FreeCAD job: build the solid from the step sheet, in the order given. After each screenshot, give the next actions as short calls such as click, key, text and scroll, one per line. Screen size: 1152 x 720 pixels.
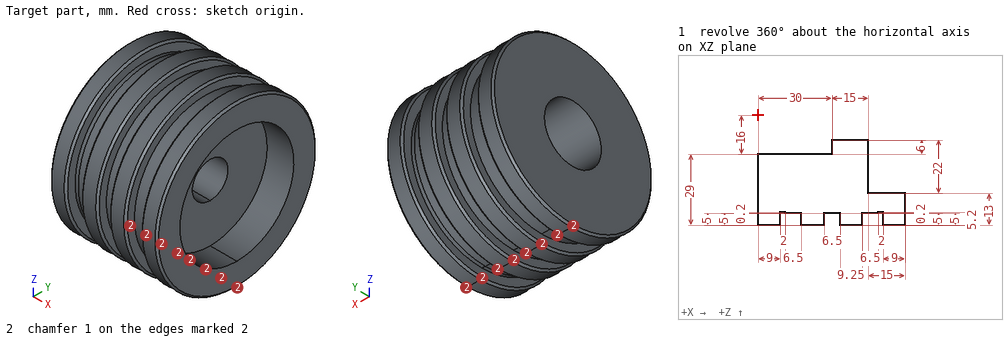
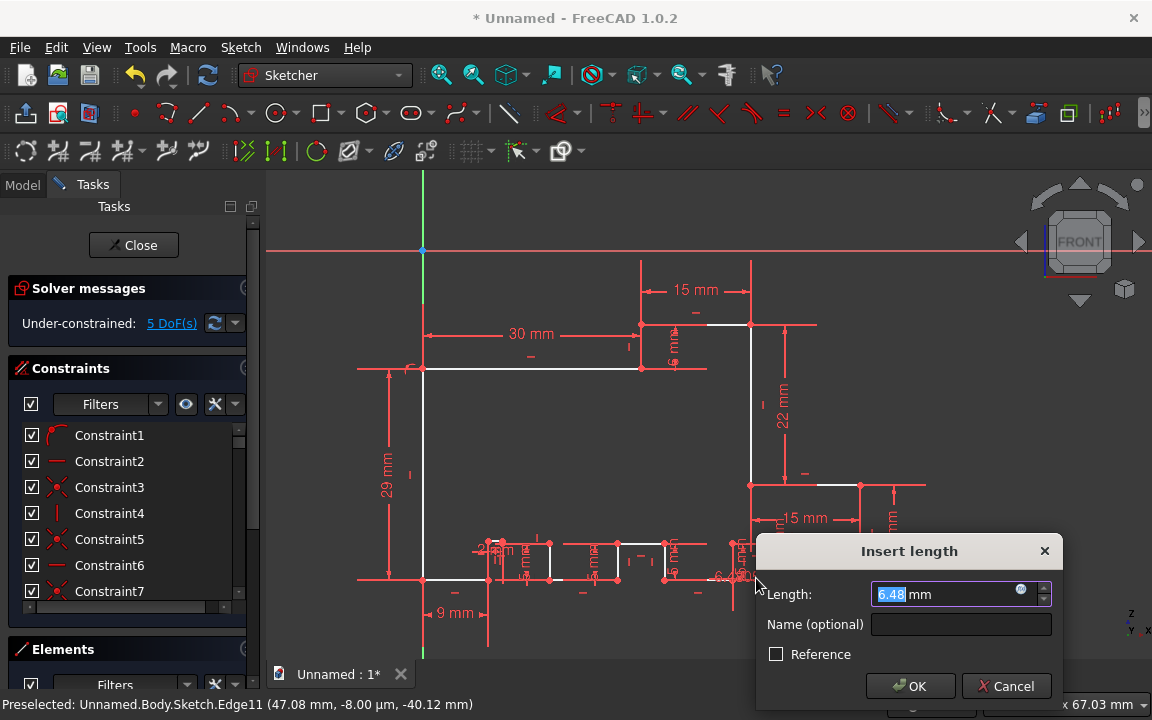
text(6.5)
key(Return)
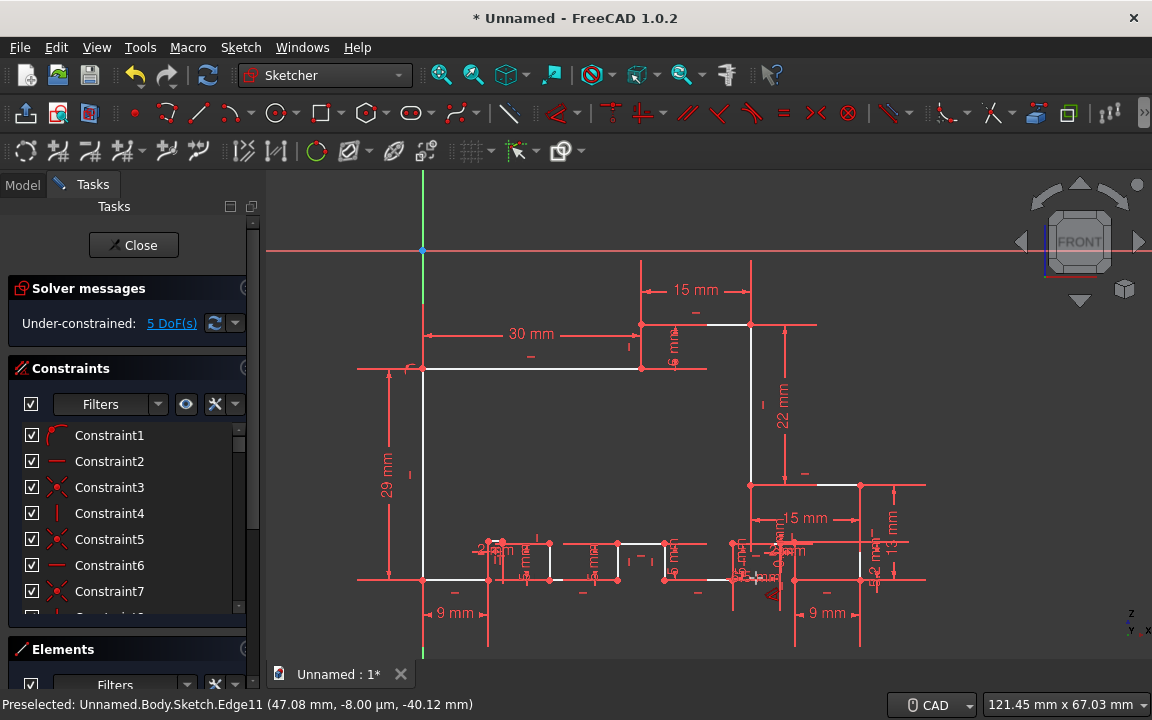
click(651, 544)
click(641, 510)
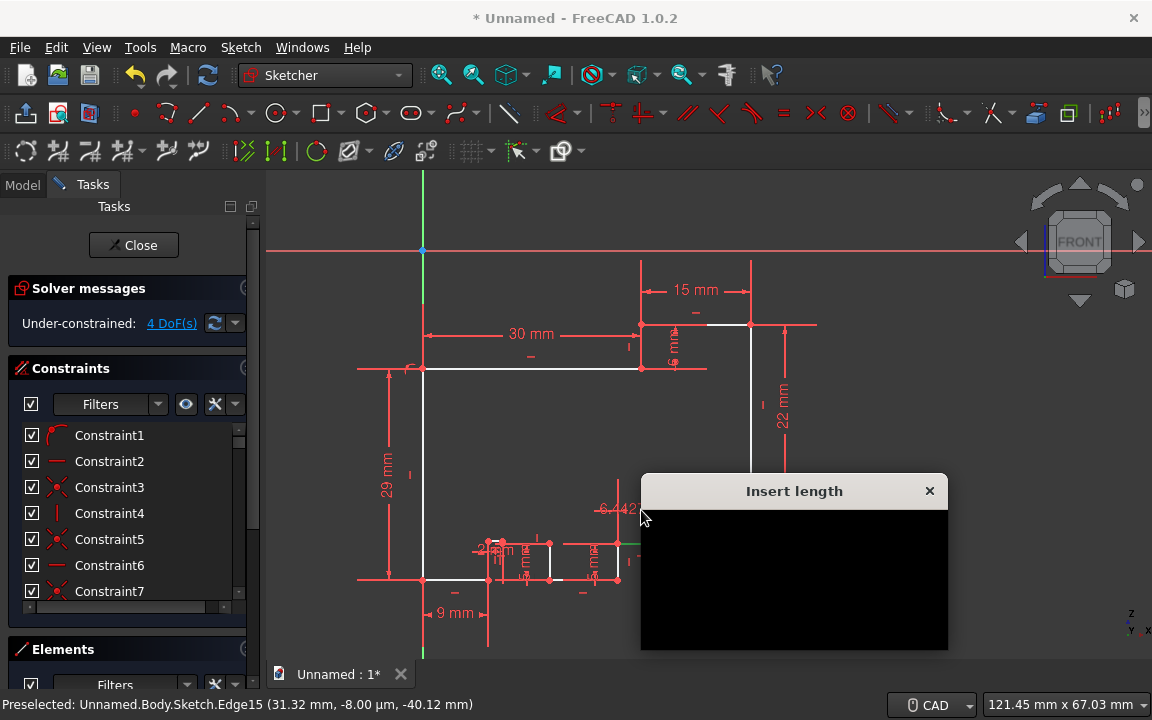
text(6.5)
key(Return)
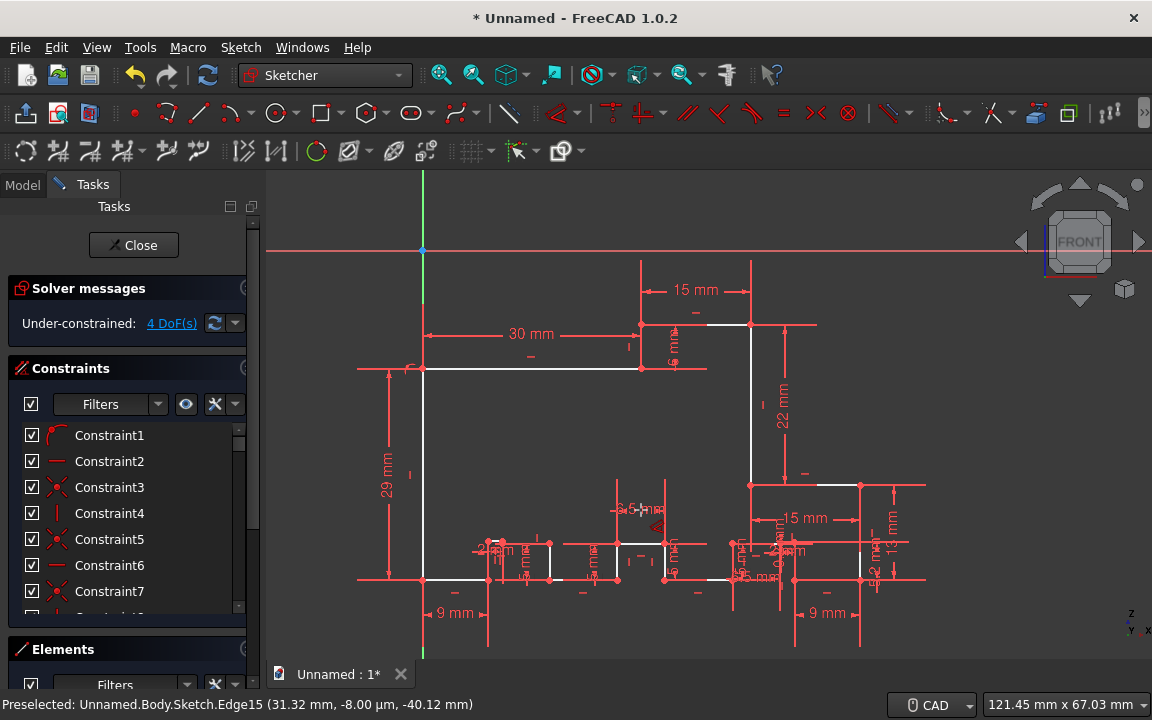
click(536, 544)
click(526, 510)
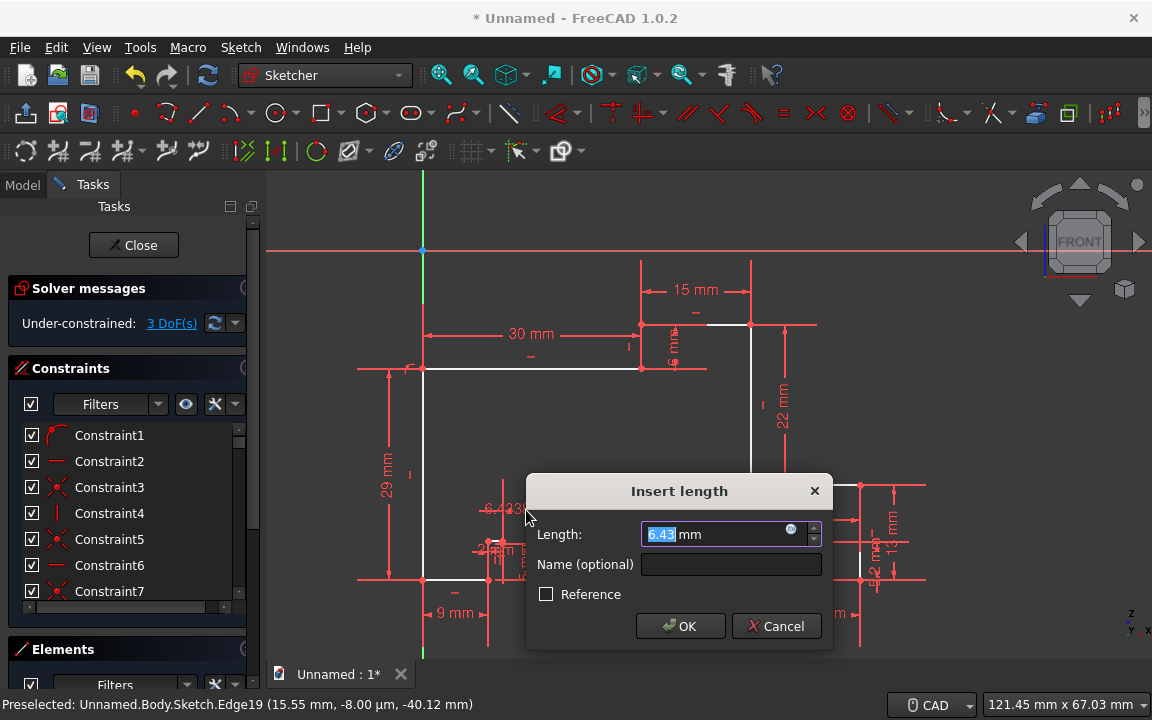
text(6.5)
key(Return)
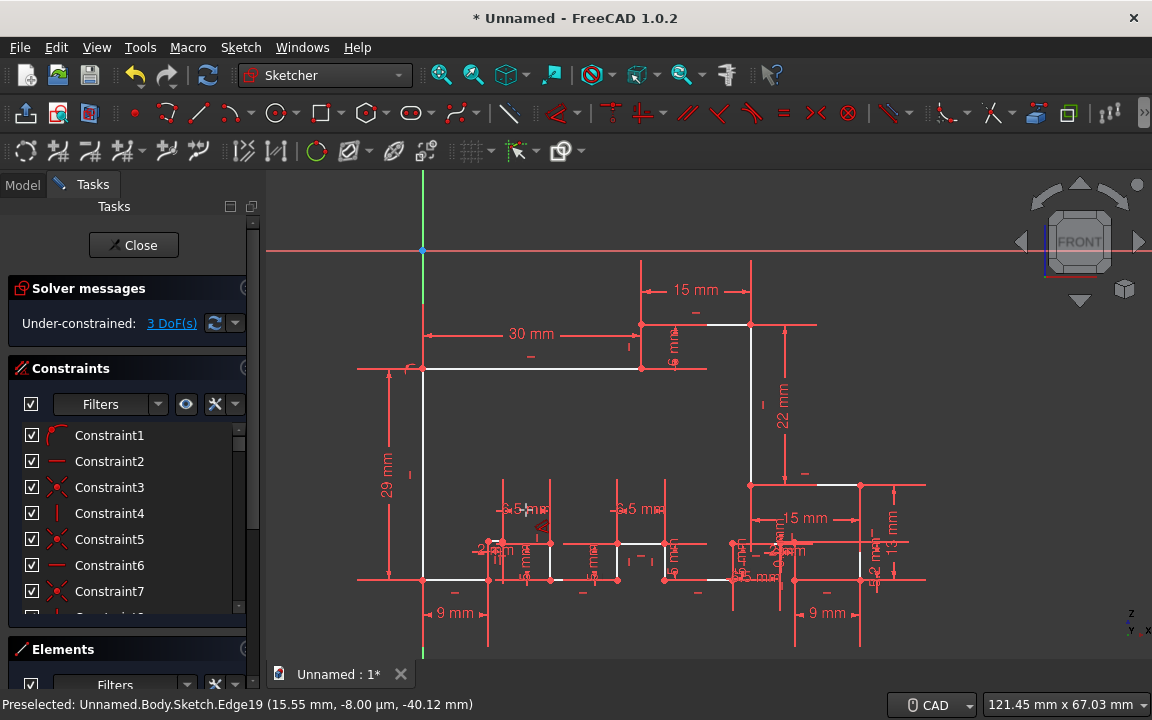
scroll(503, 542, up, 17)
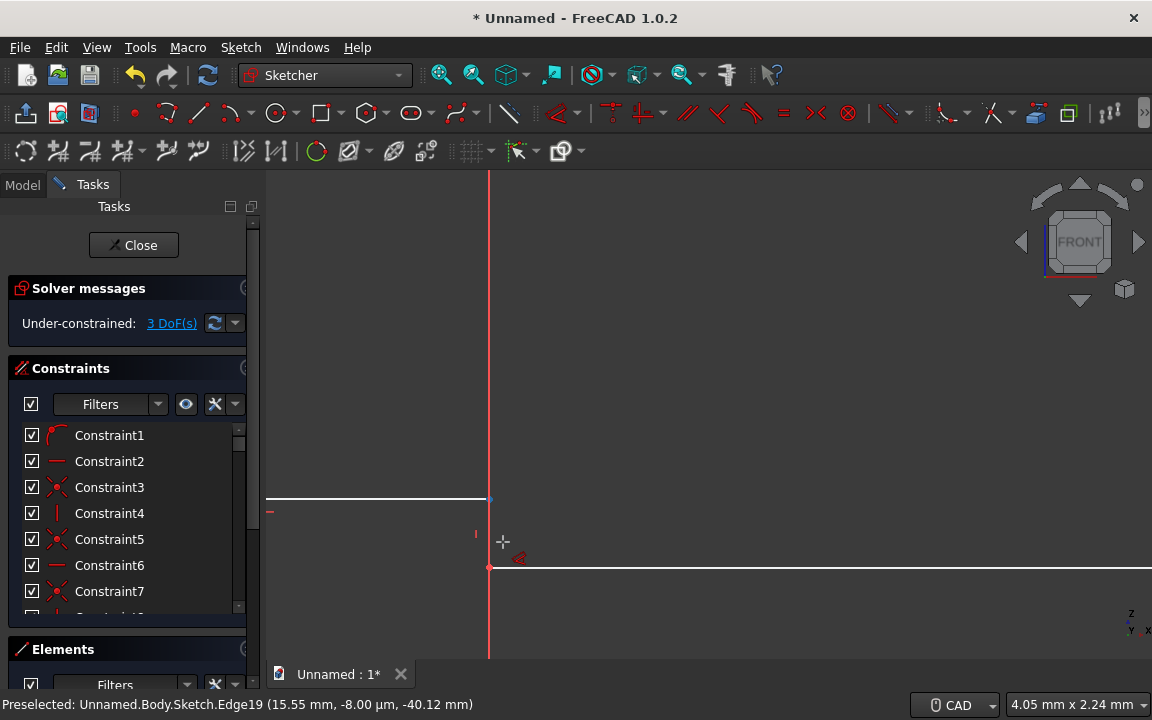
click(489, 533)
click(455, 533)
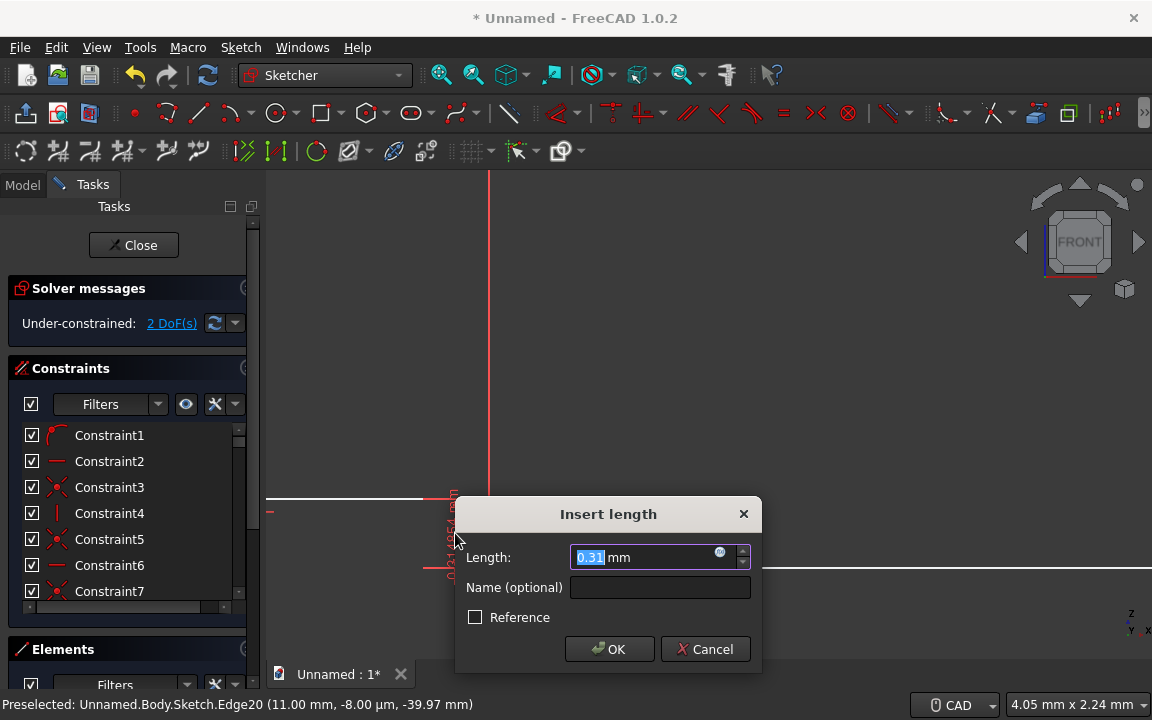
text(0.2)
key(Return)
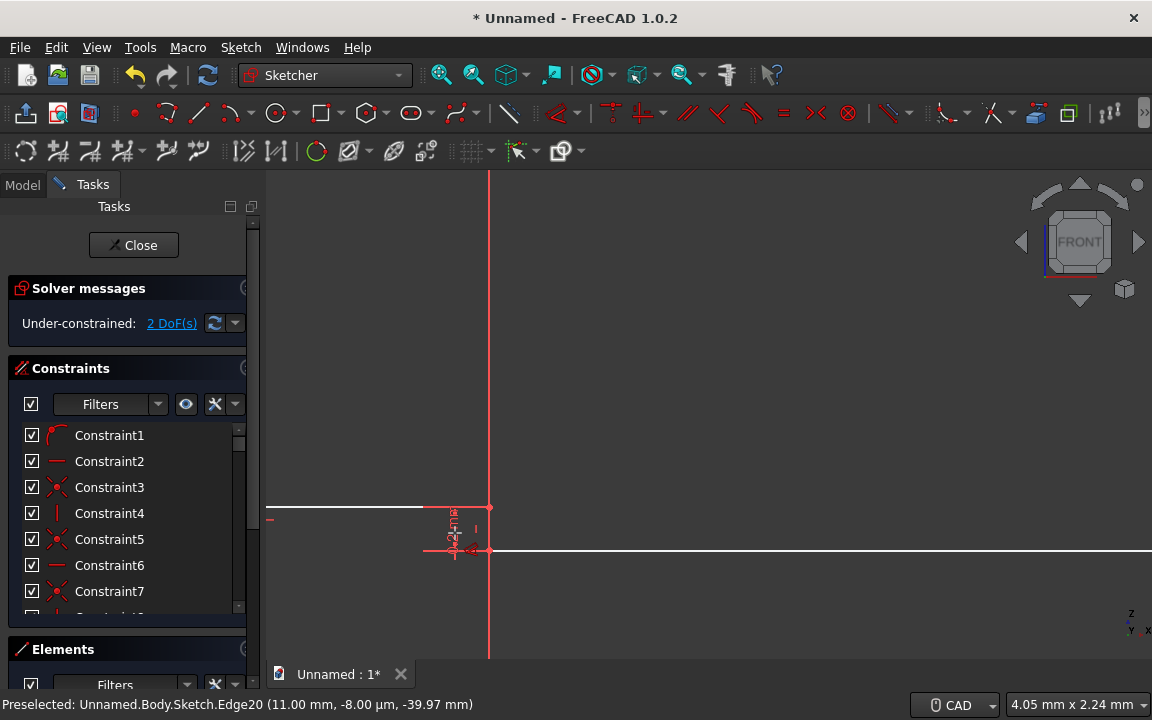
scroll(502, 542, down, 17)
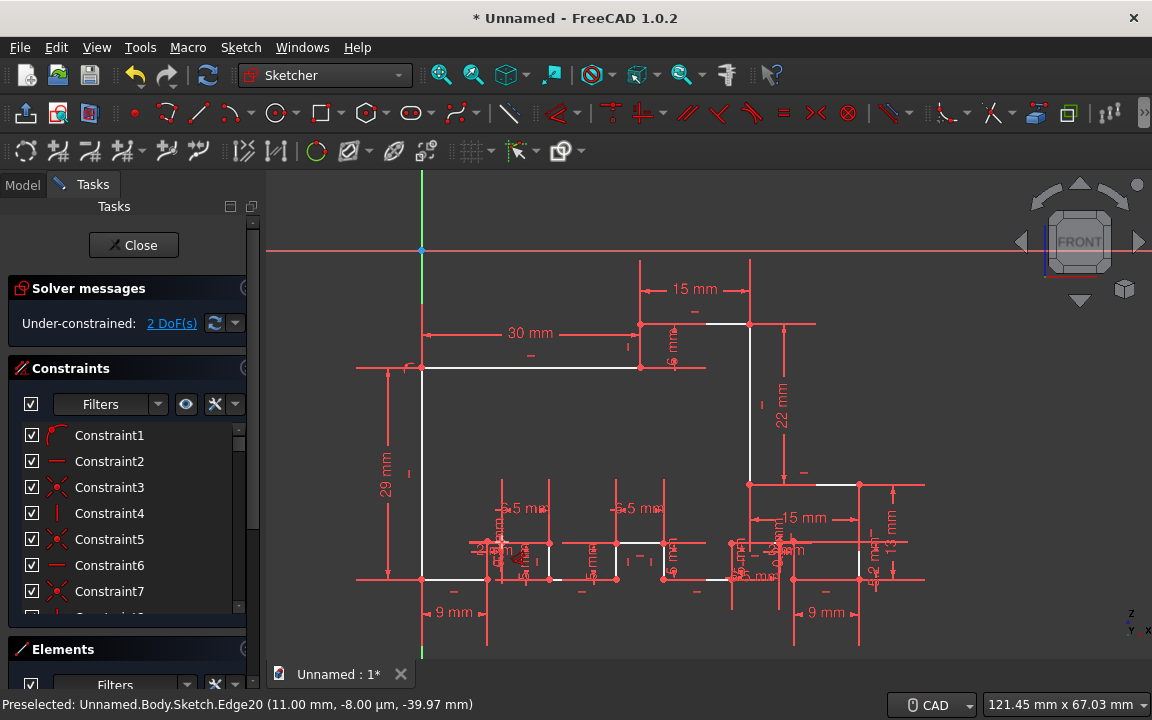
click(422, 368)
click(388, 309)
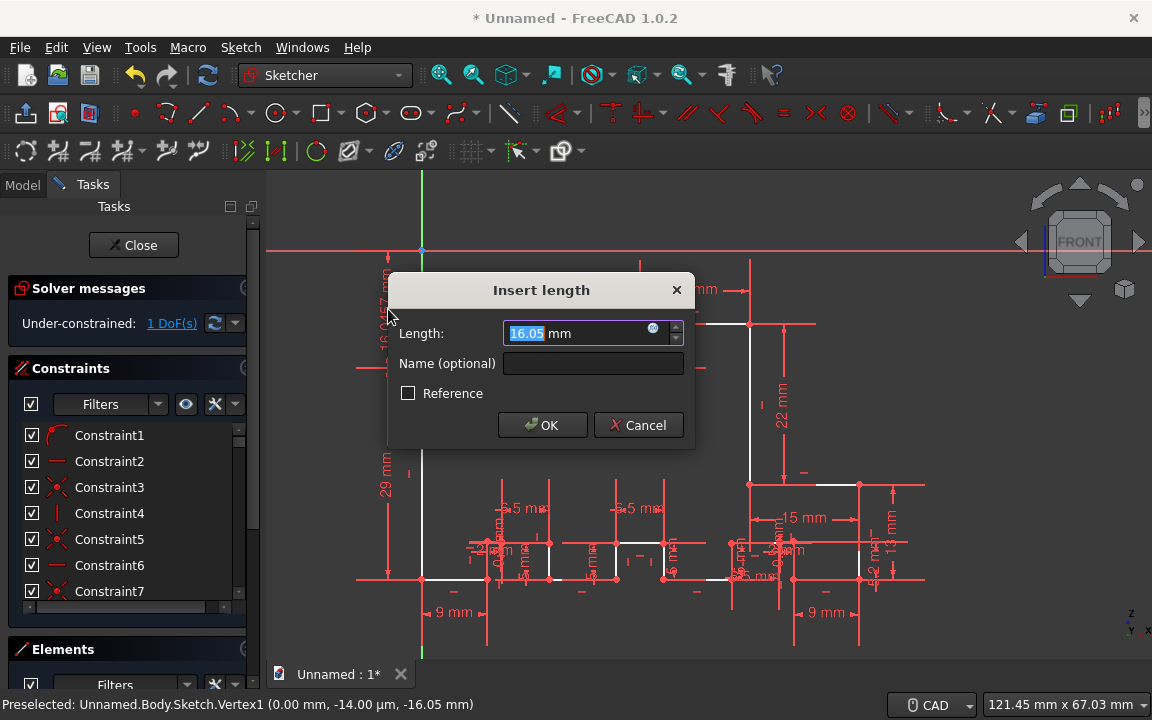
text(16)
key(Return)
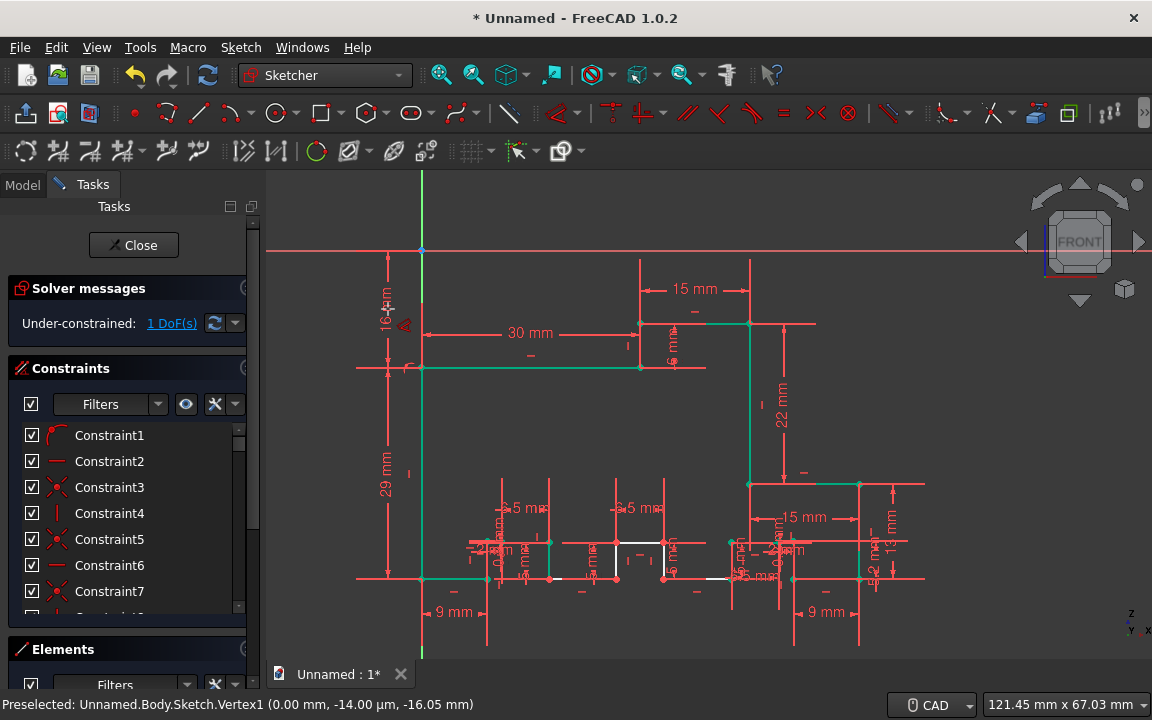
click(711, 579)
click(698, 613)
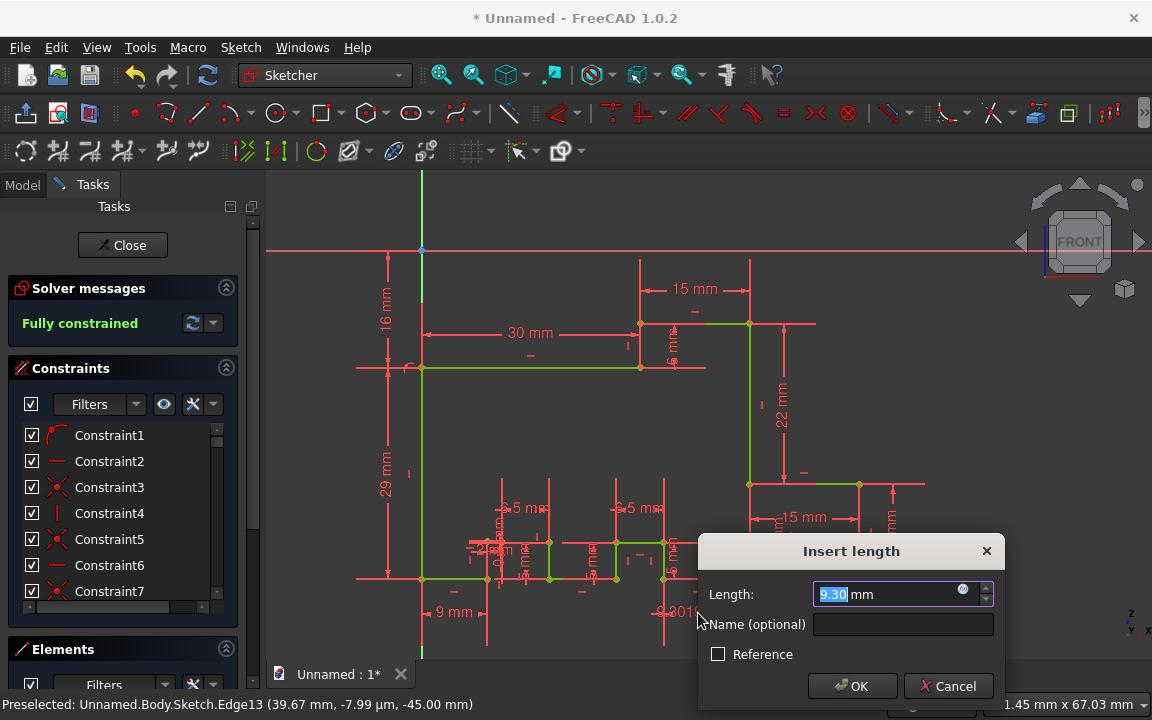
text(9.25)
key(Return)
key(Escape)